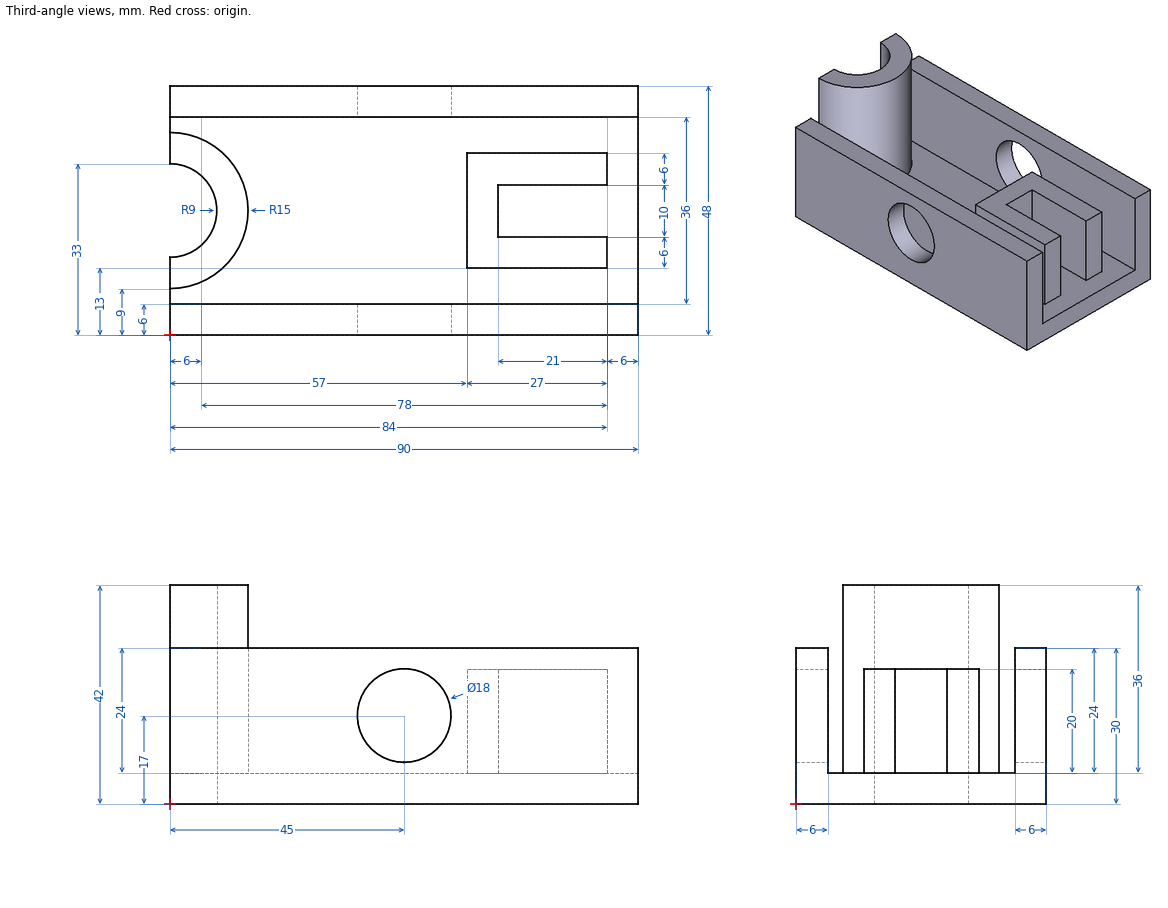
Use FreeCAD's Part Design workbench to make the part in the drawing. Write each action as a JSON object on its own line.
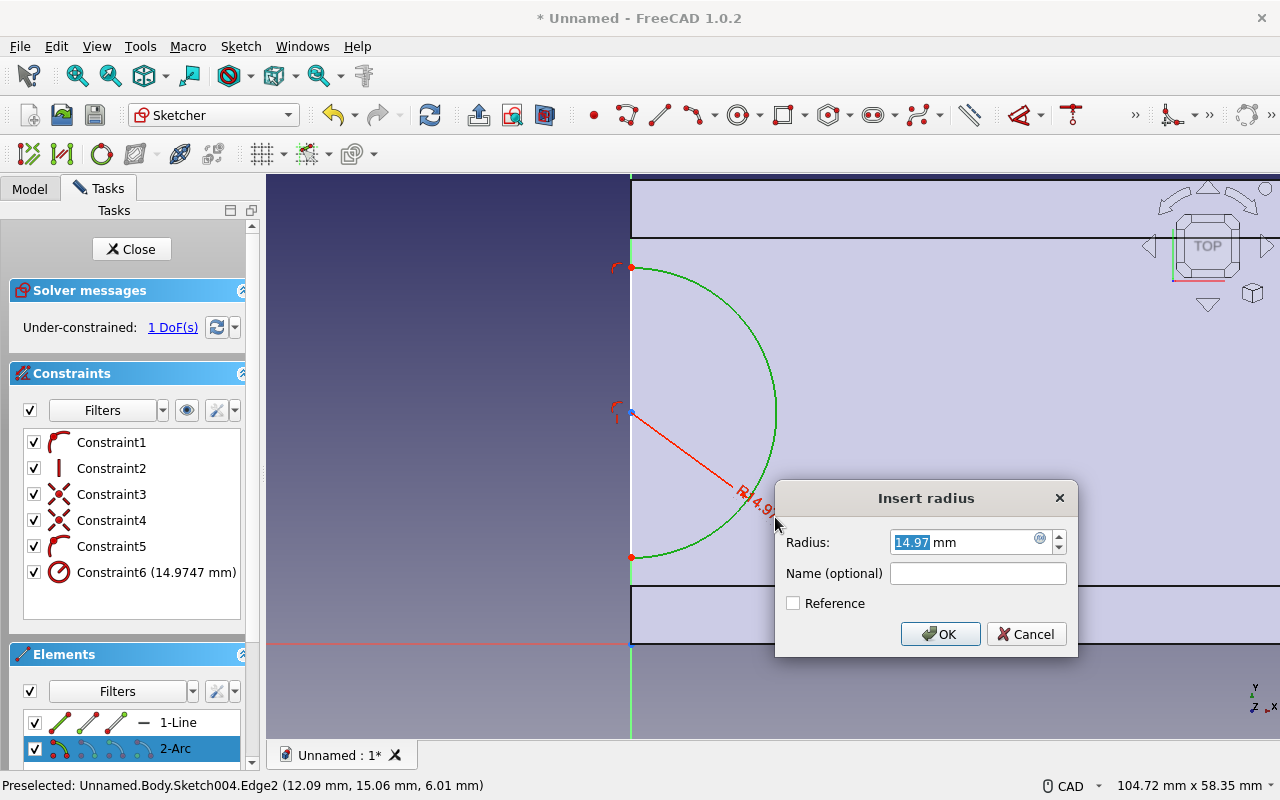
{"action": "type", "text": "15"}
{"action": "key", "text": "Return"}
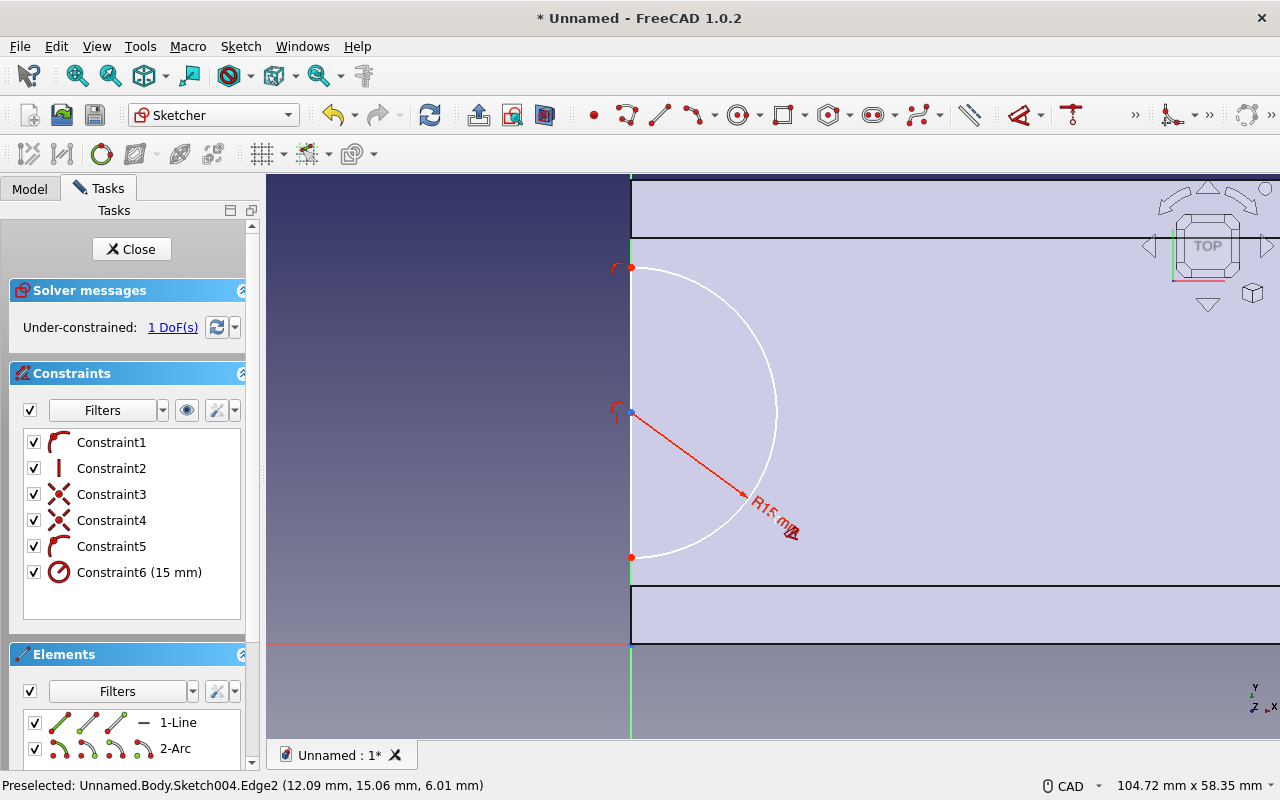
{"action": "left_click", "coordinate": [631, 558]}
{"action": "left_click", "coordinate": [597, 601]}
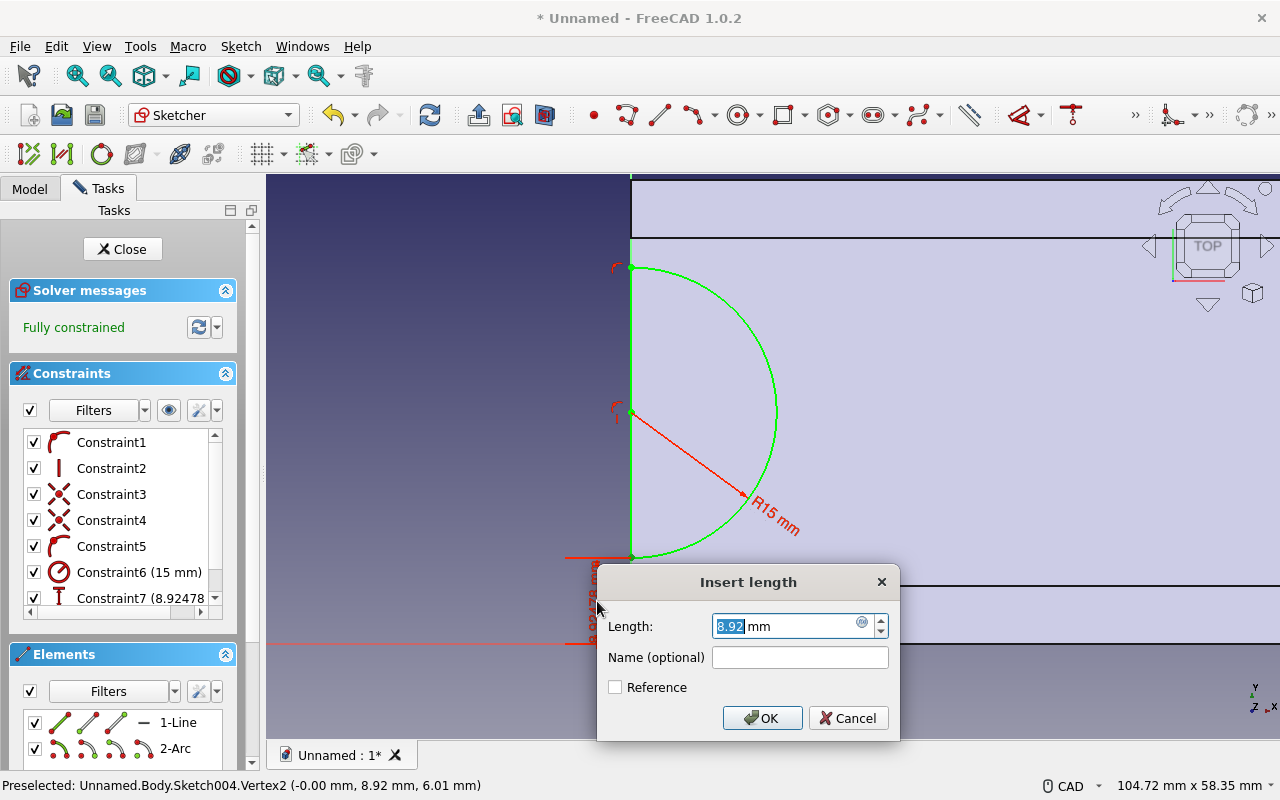
{"action": "type", "text": "9"}
{"action": "key", "text": "Return"}
{"action": "key", "text": "Escape"}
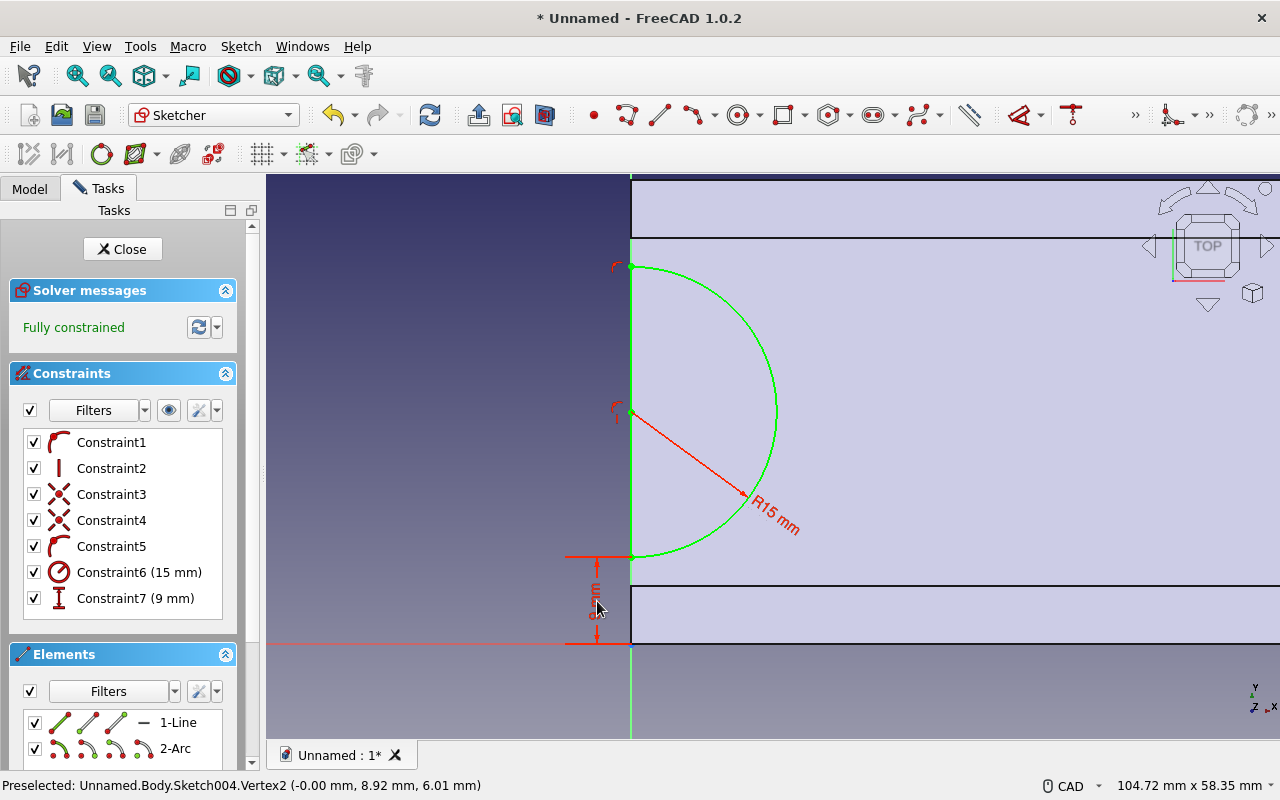
{"action": "left_click", "coordinate": [123, 249]}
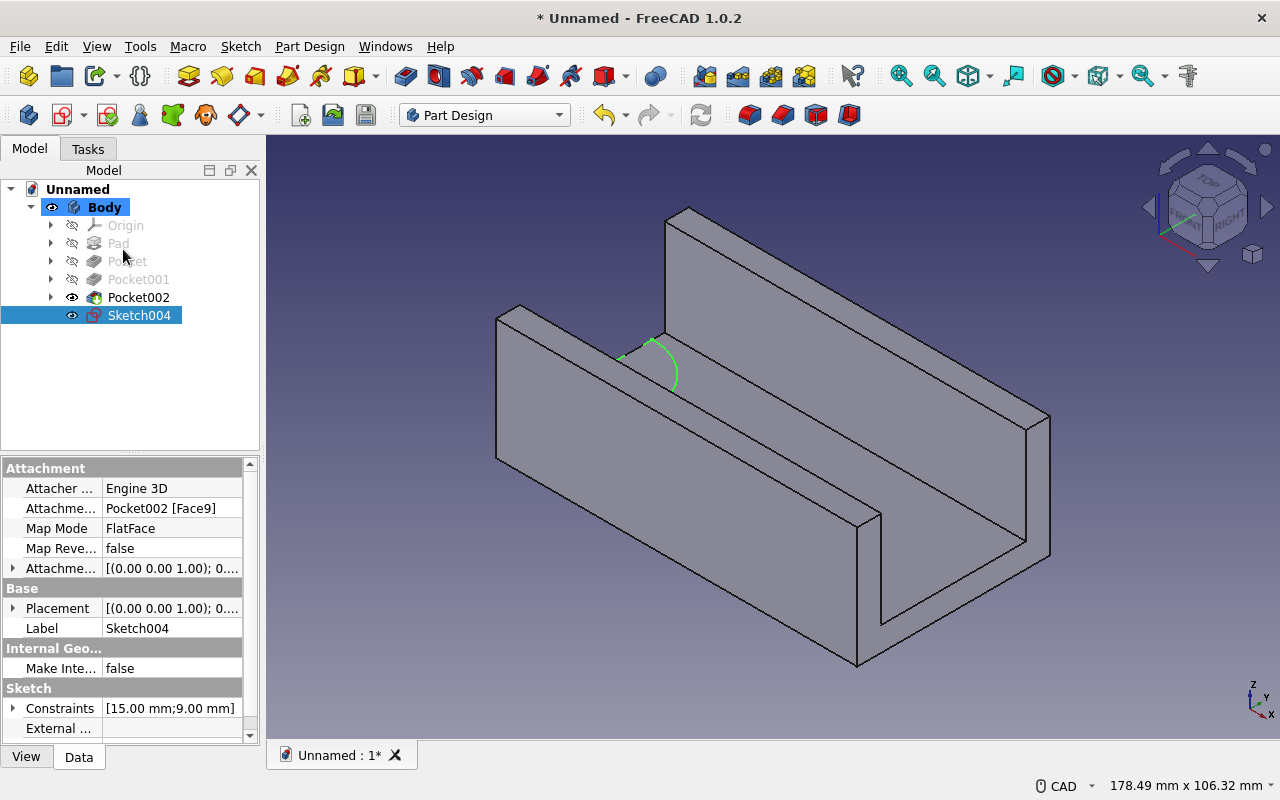
{"action": "left_click", "coordinate": [189, 76]}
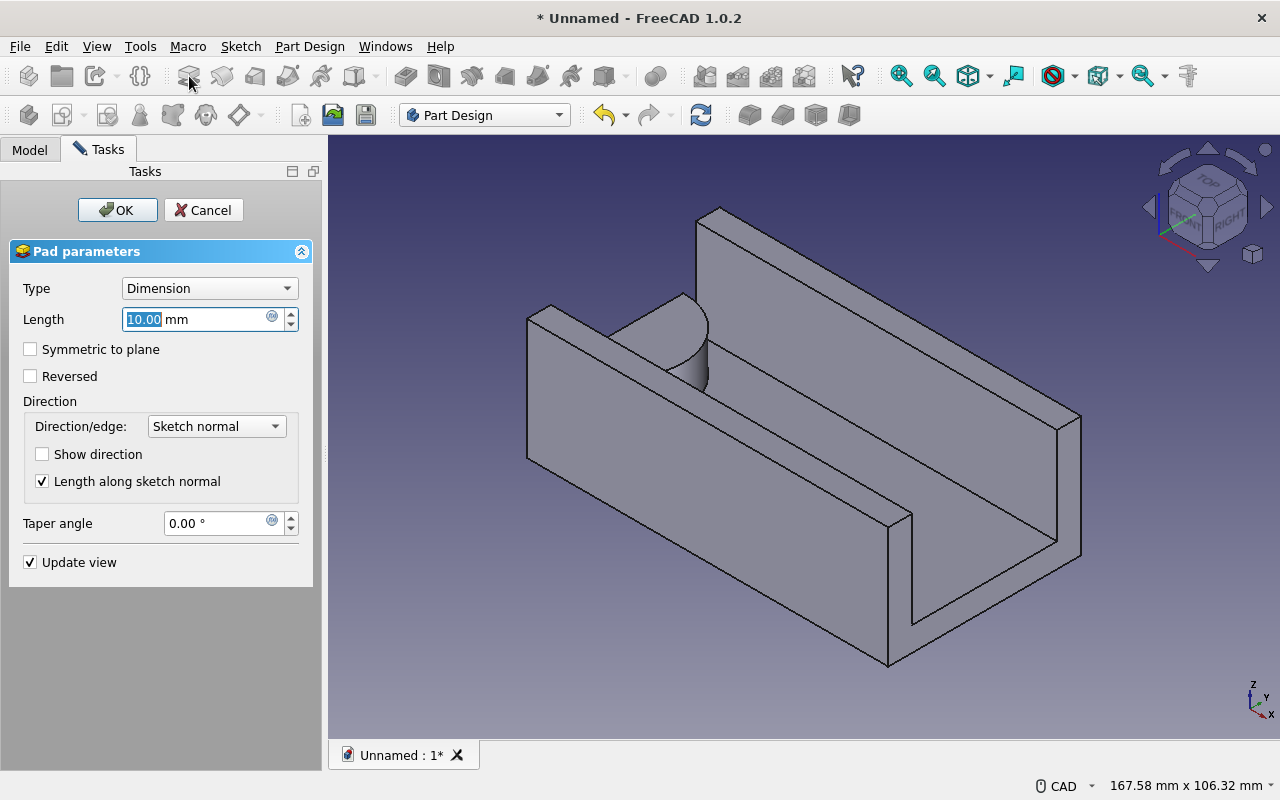
{"action": "type", "text": "36"}
{"action": "key", "text": "Tab"}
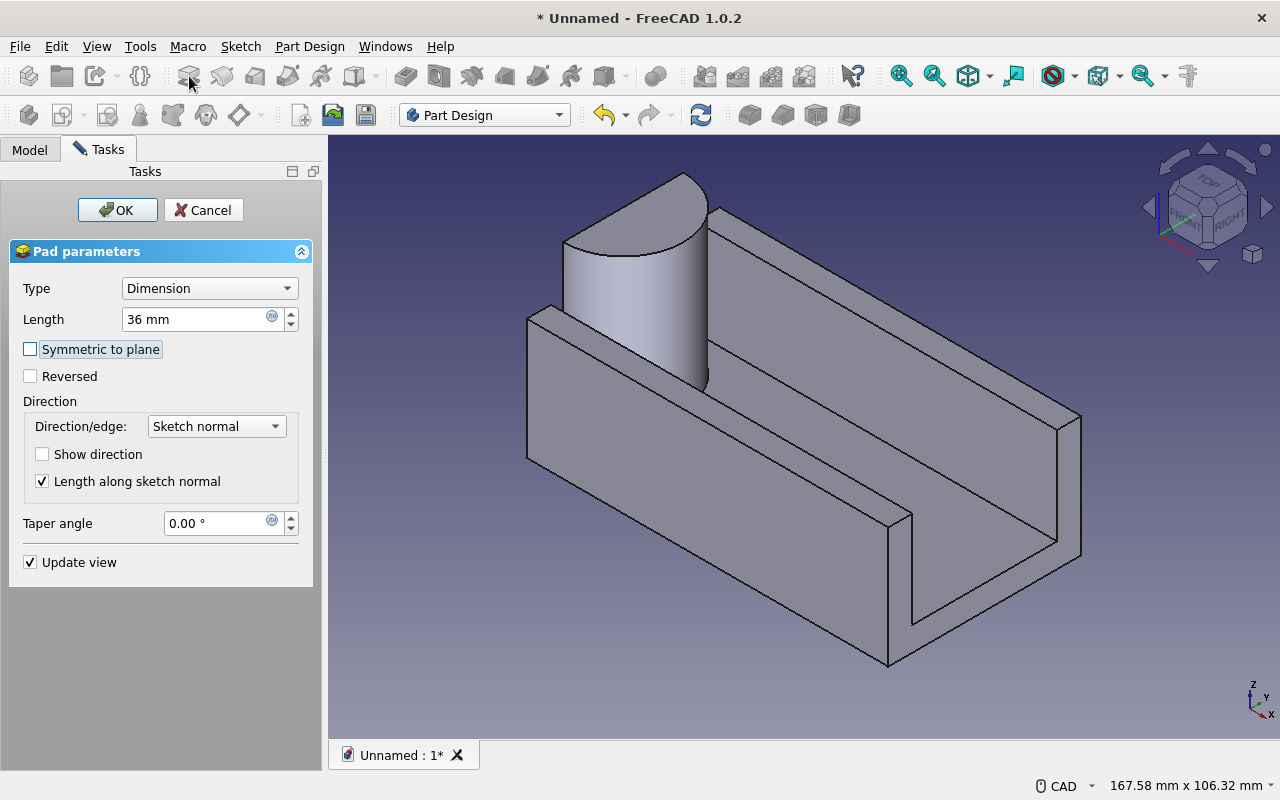
{"action": "left_click", "coordinate": [118, 210]}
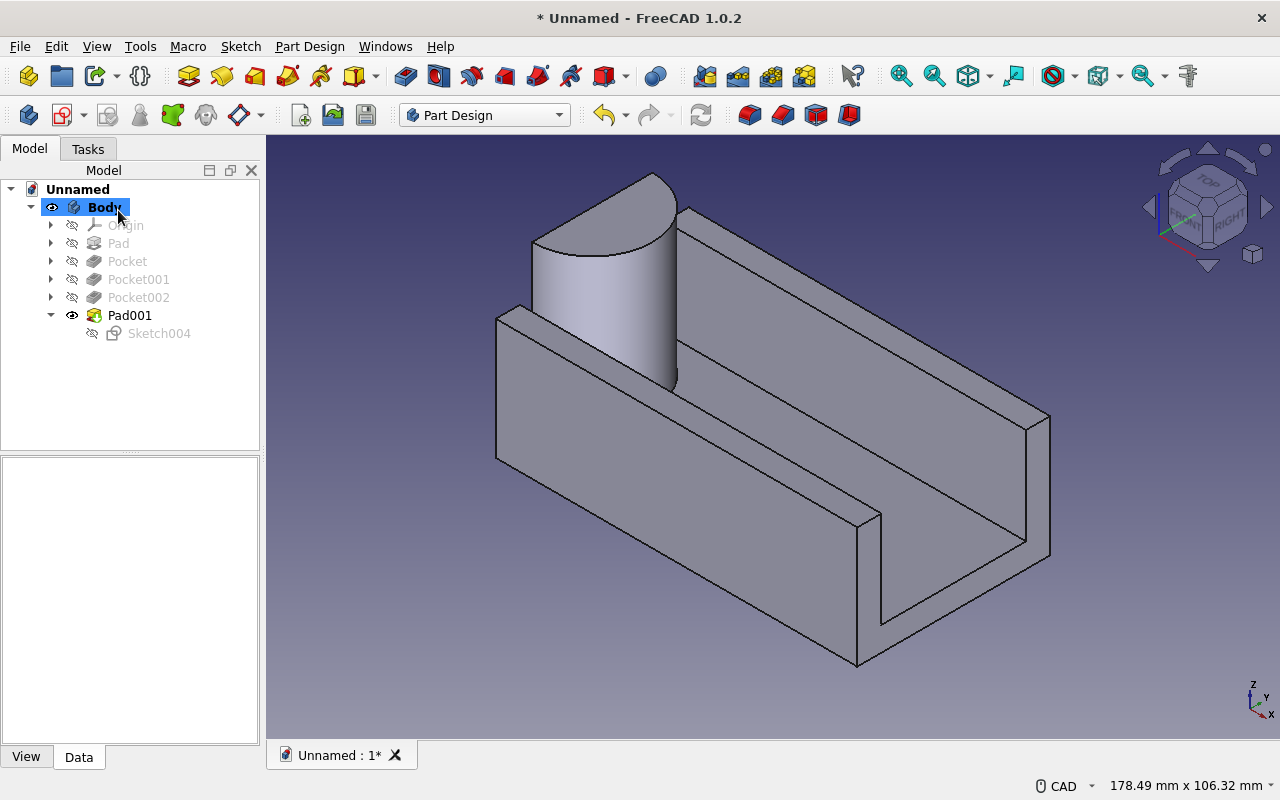
{"action": "left_click", "coordinate": [622, 224]}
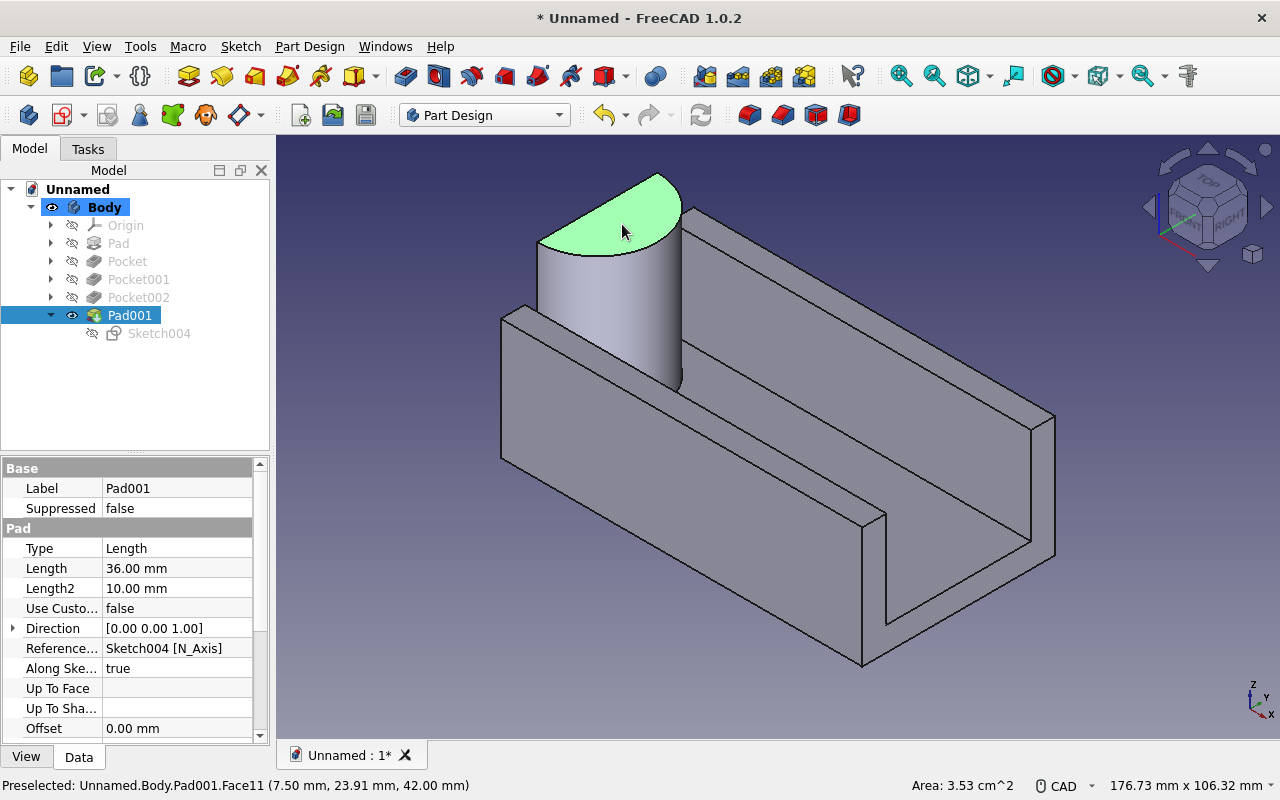
{"action": "left_click", "coordinate": [62, 116]}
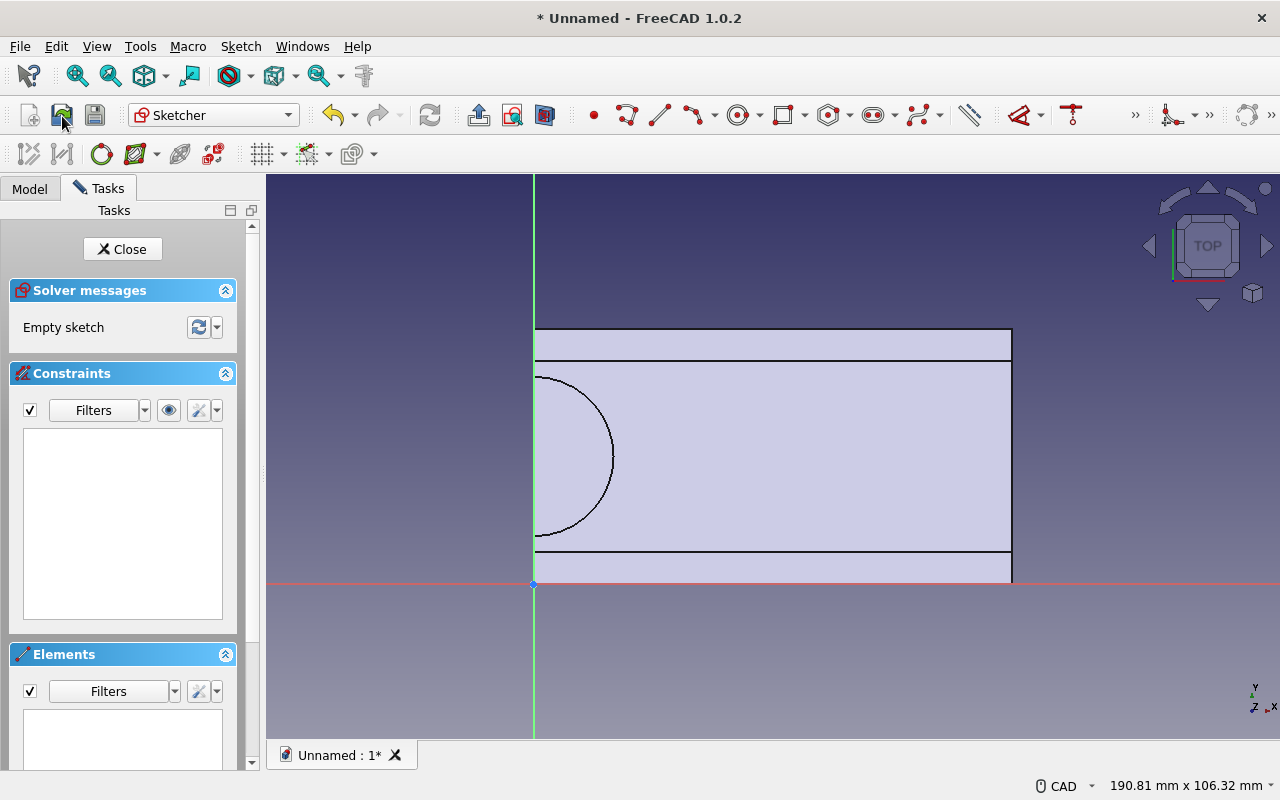
{"action": "scroll", "coordinate": [438, 529], "scroll_direction": "up", "scroll_amount": 4}